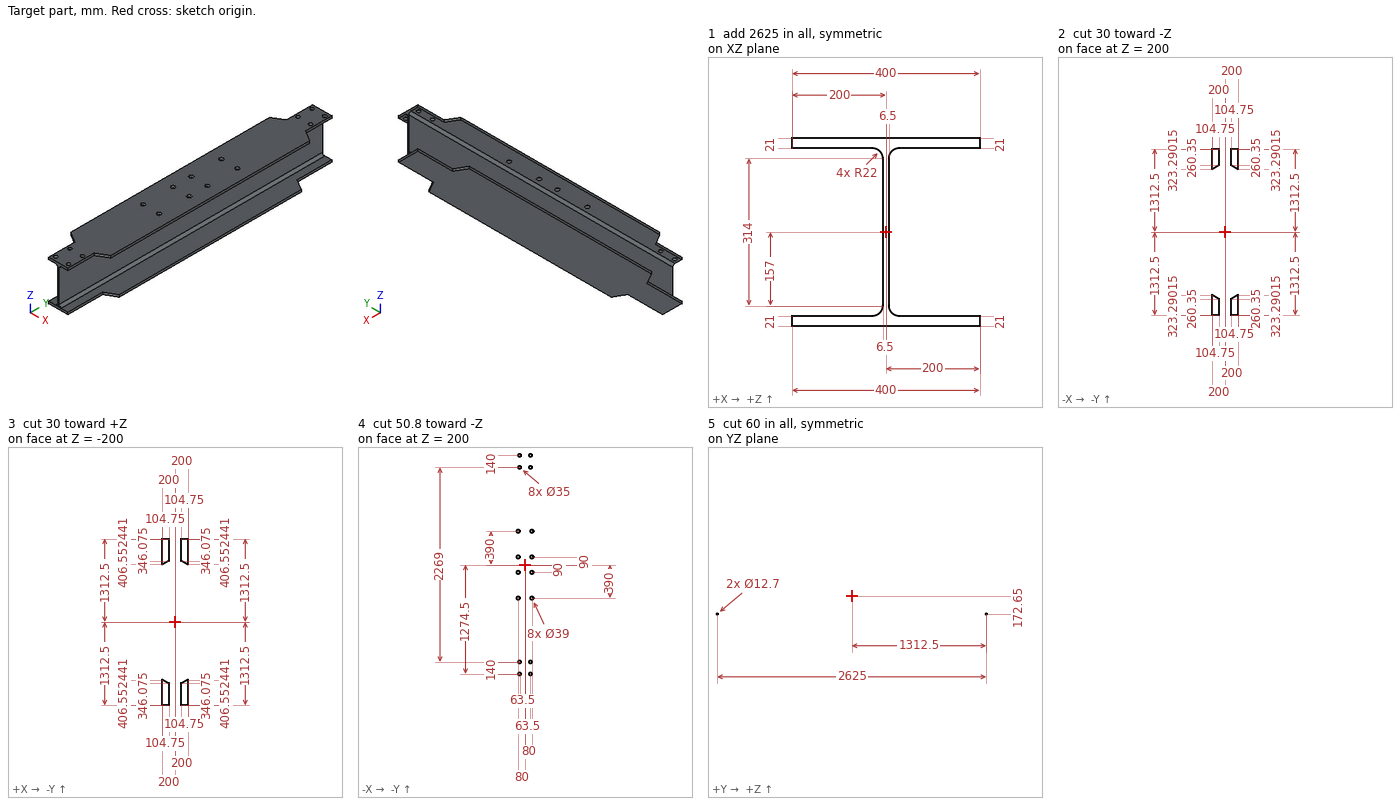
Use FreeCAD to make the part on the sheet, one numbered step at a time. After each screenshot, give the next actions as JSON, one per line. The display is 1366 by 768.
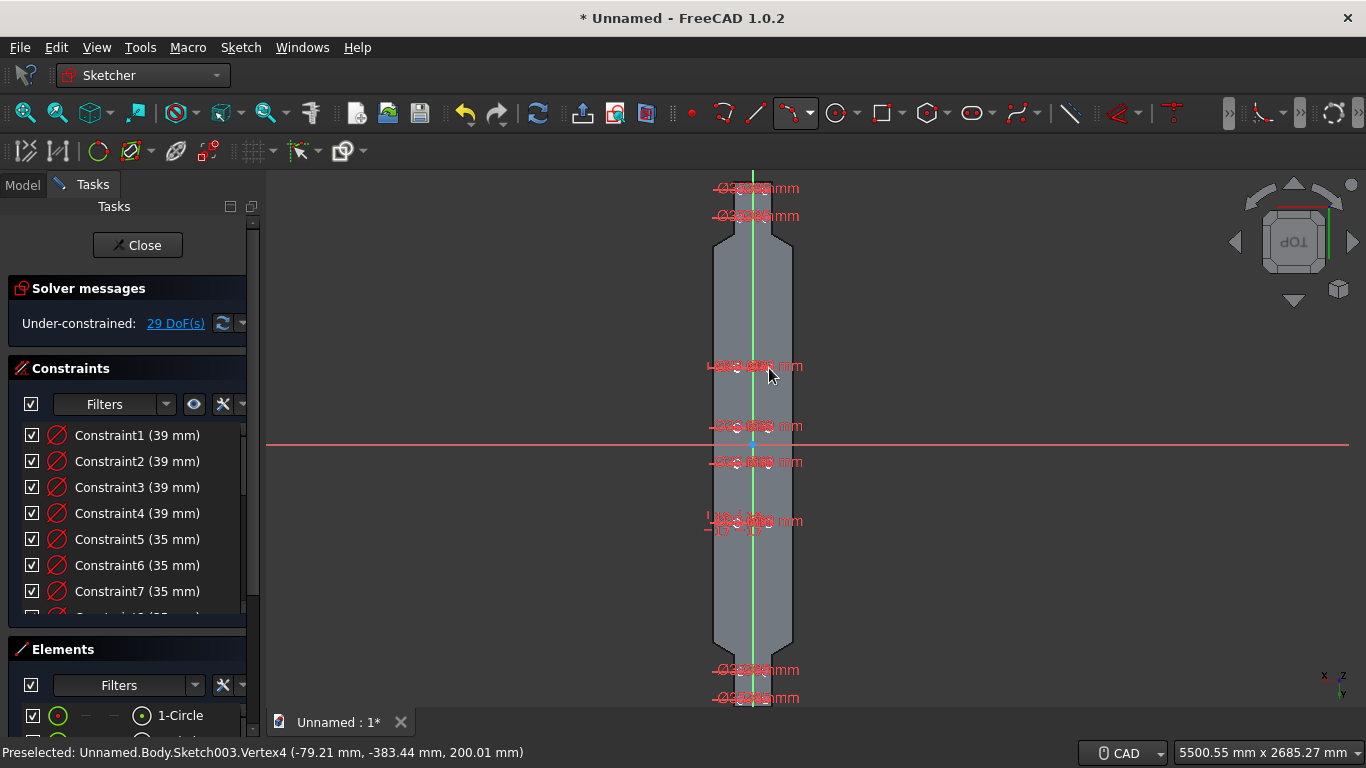
{"action": "scroll", "coordinate": [737, 368], "scroll_direction": "up", "scroll_amount": 4}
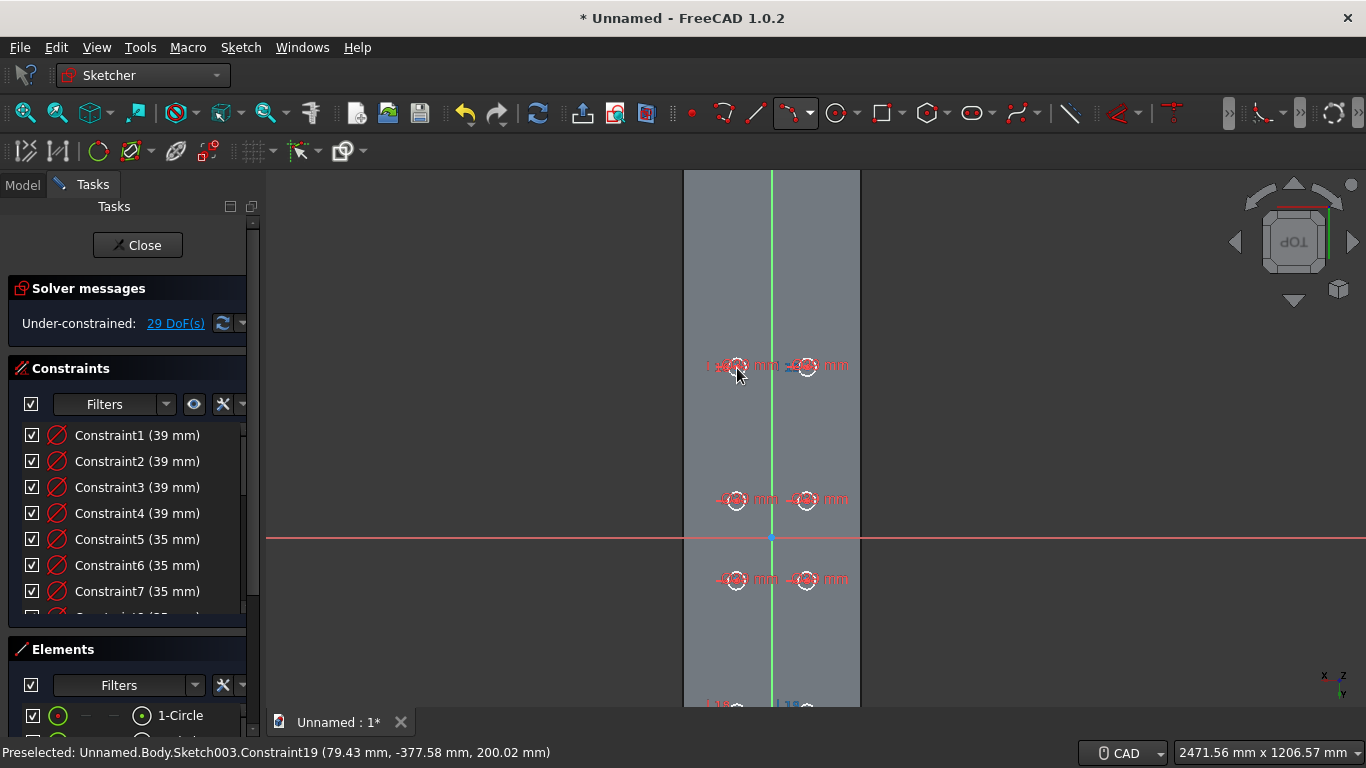
{"action": "left_click", "coordinate": [737, 367]}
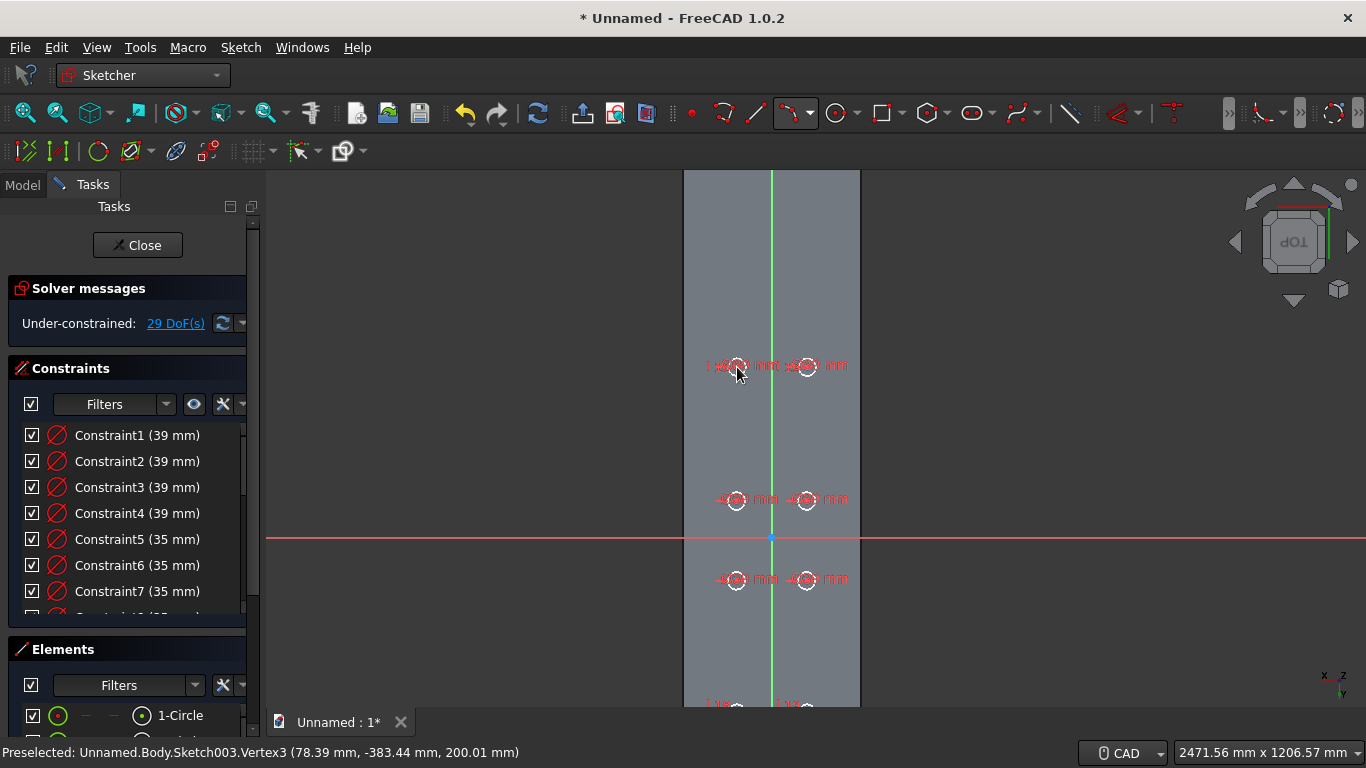
{"action": "left_click", "coordinate": [807, 367]}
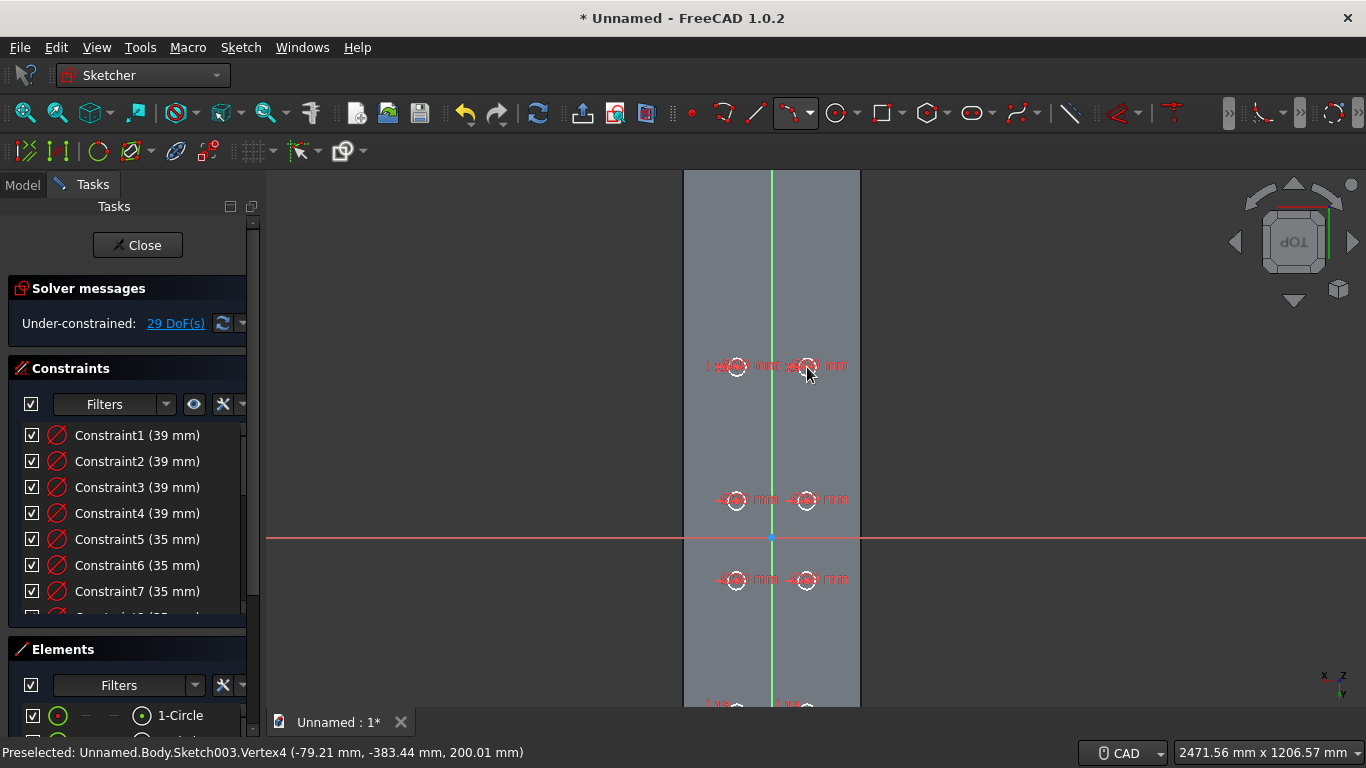
{"action": "key", "text": "h"}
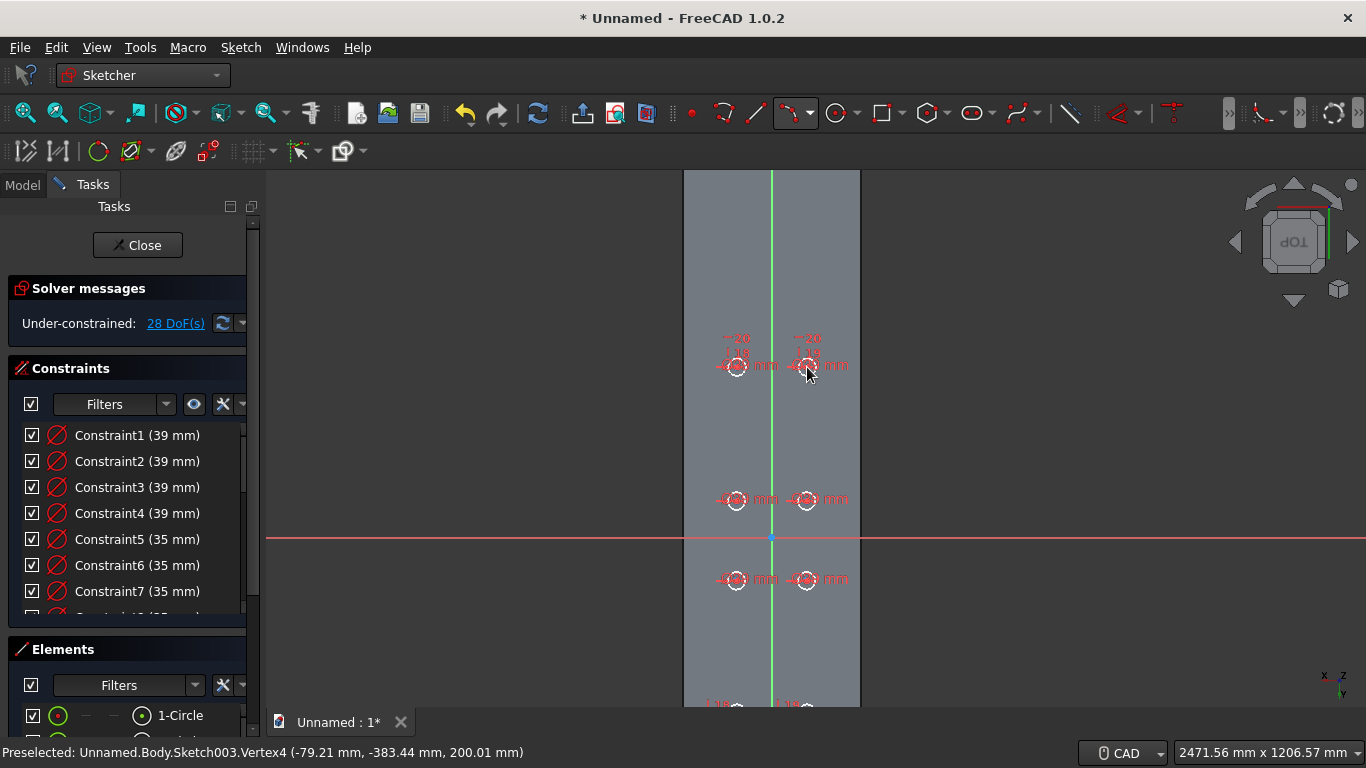
{"action": "scroll", "coordinate": [737, 396], "scroll_direction": "down", "scroll_amount": 6}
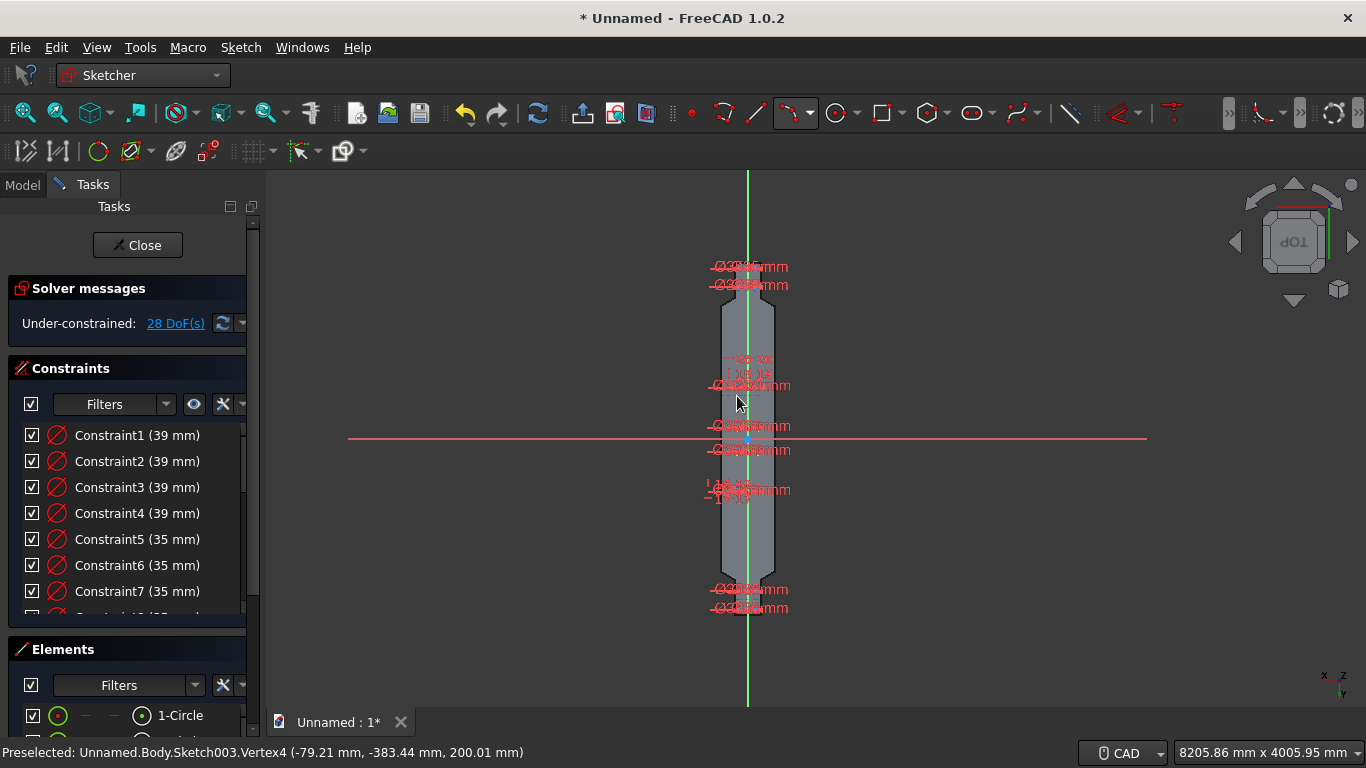
{"action": "left_click", "coordinate": [739, 610]}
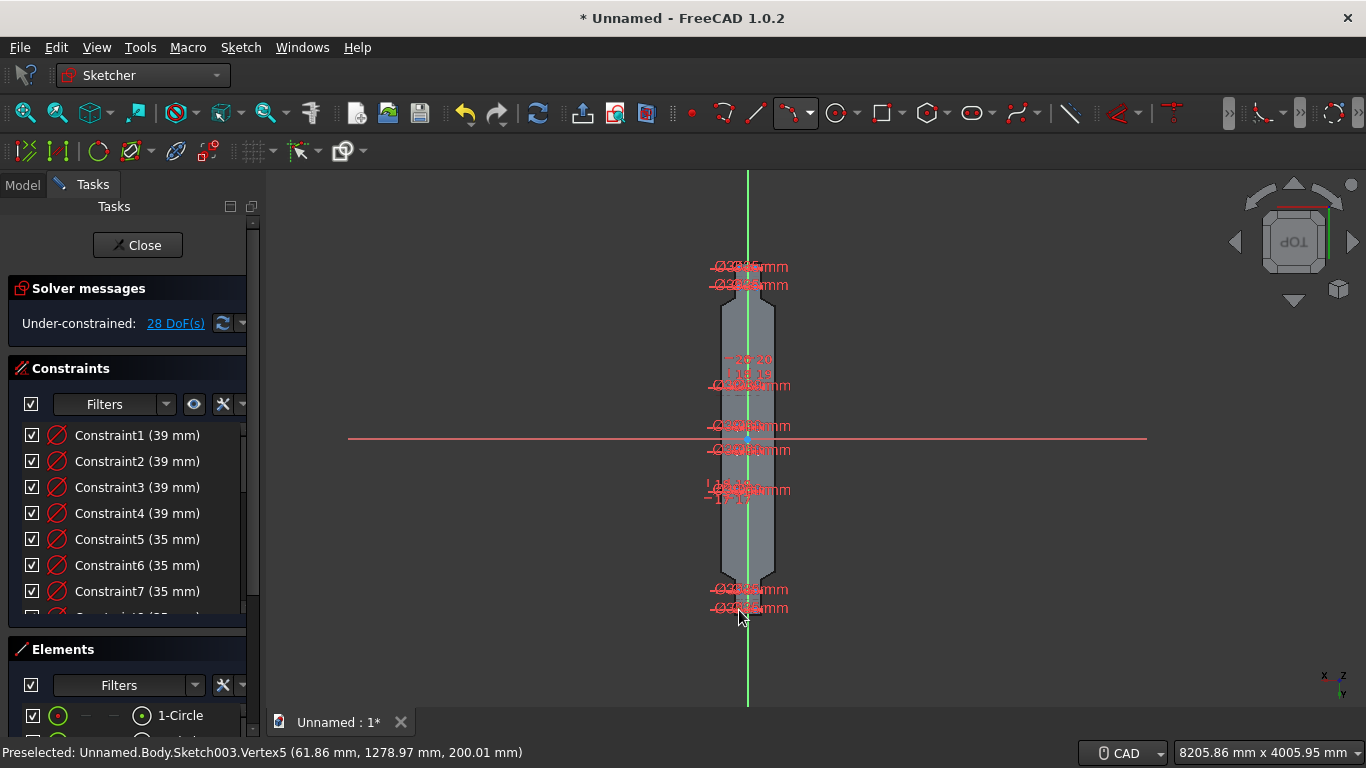
{"action": "left_click", "coordinate": [739, 591]}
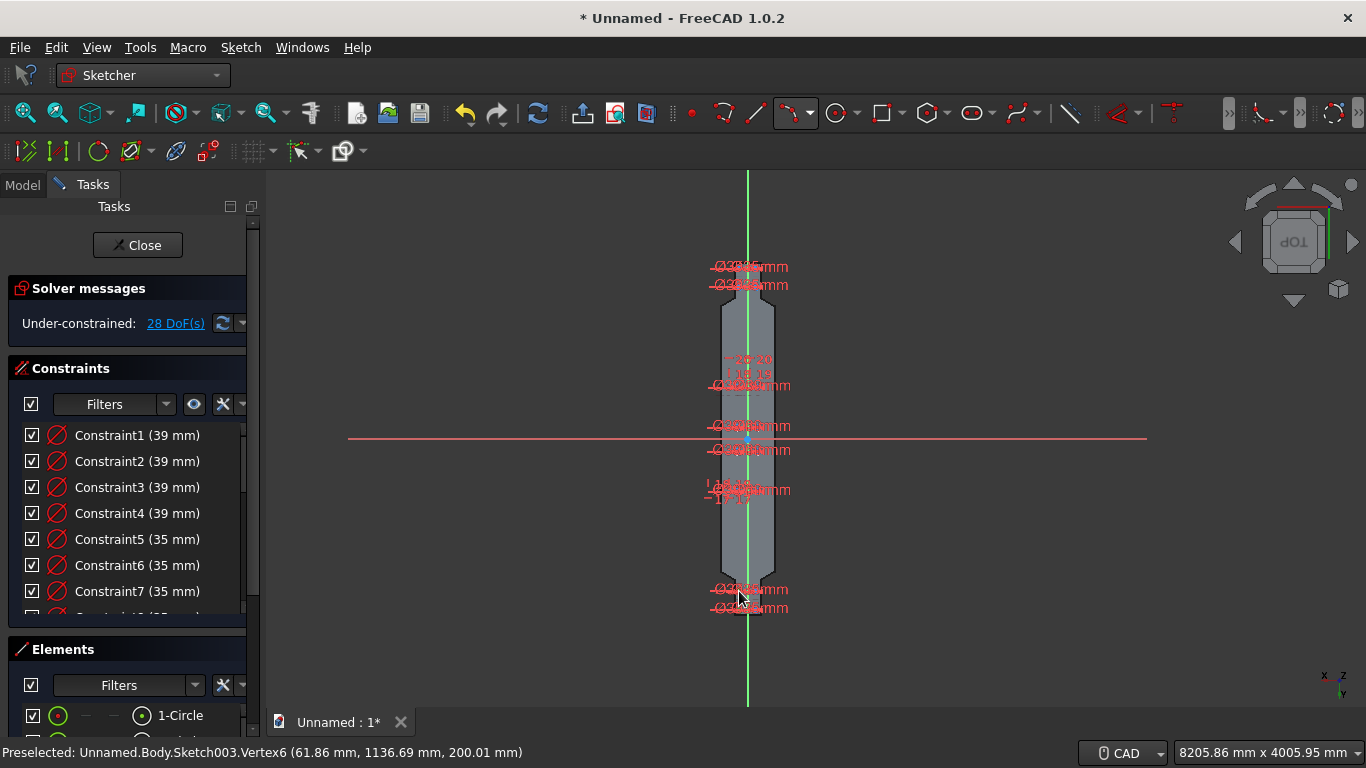
{"action": "key", "text": "v"}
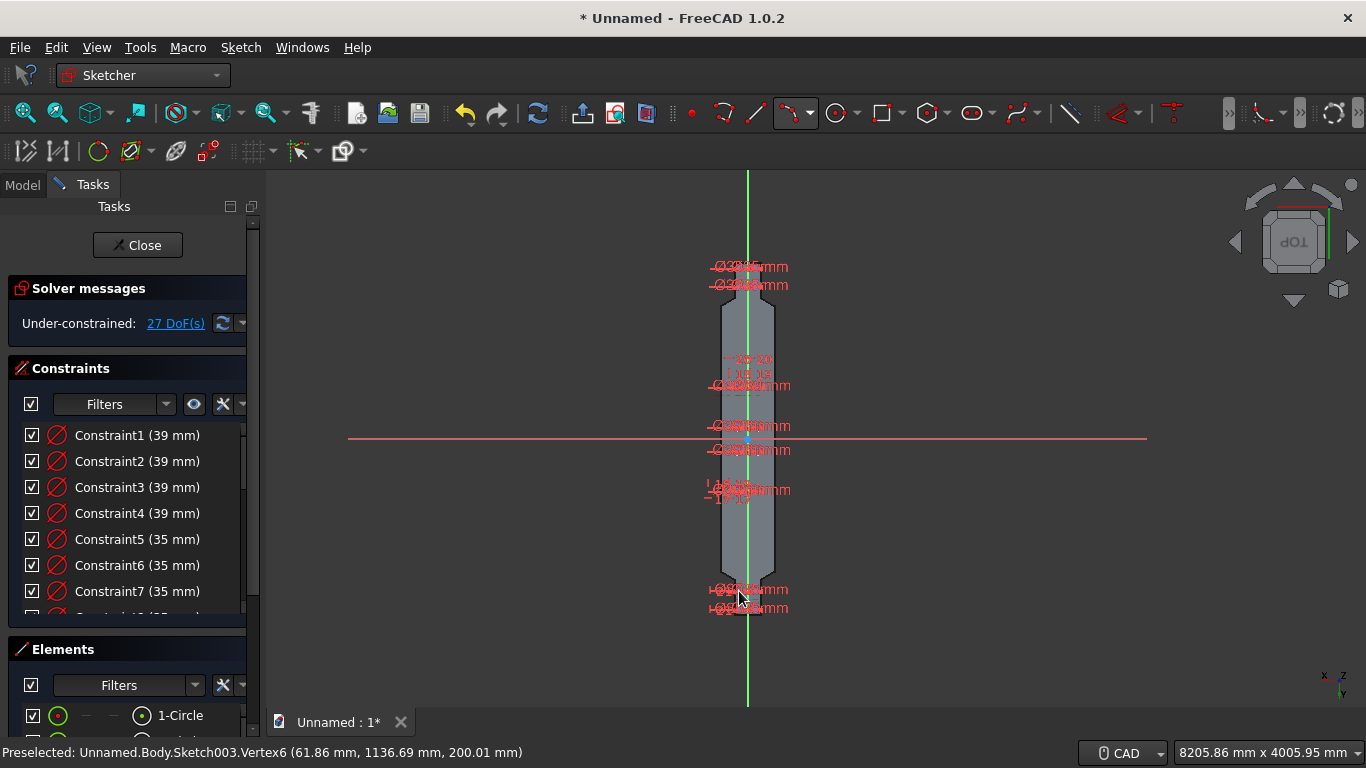
{"action": "left_click", "coordinate": [739, 610]}